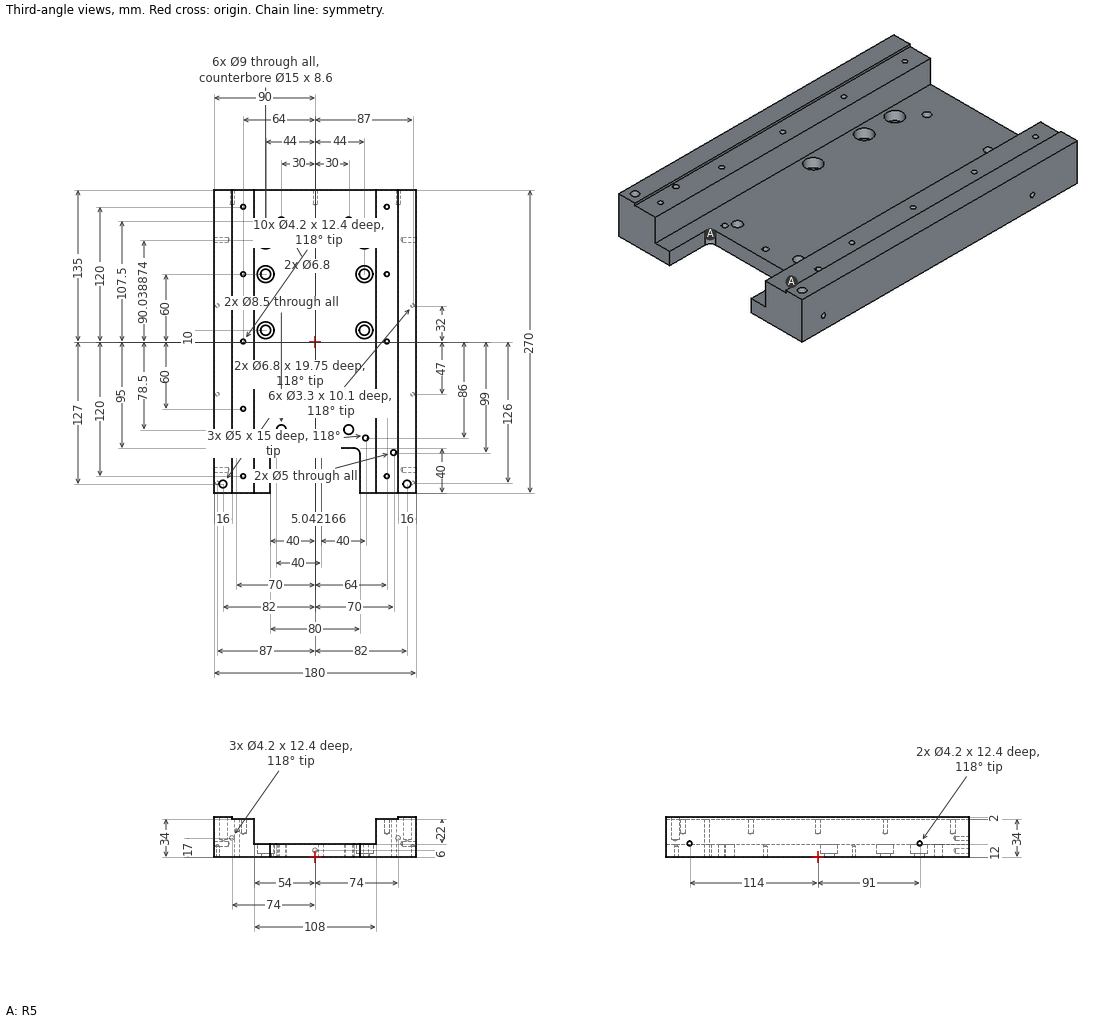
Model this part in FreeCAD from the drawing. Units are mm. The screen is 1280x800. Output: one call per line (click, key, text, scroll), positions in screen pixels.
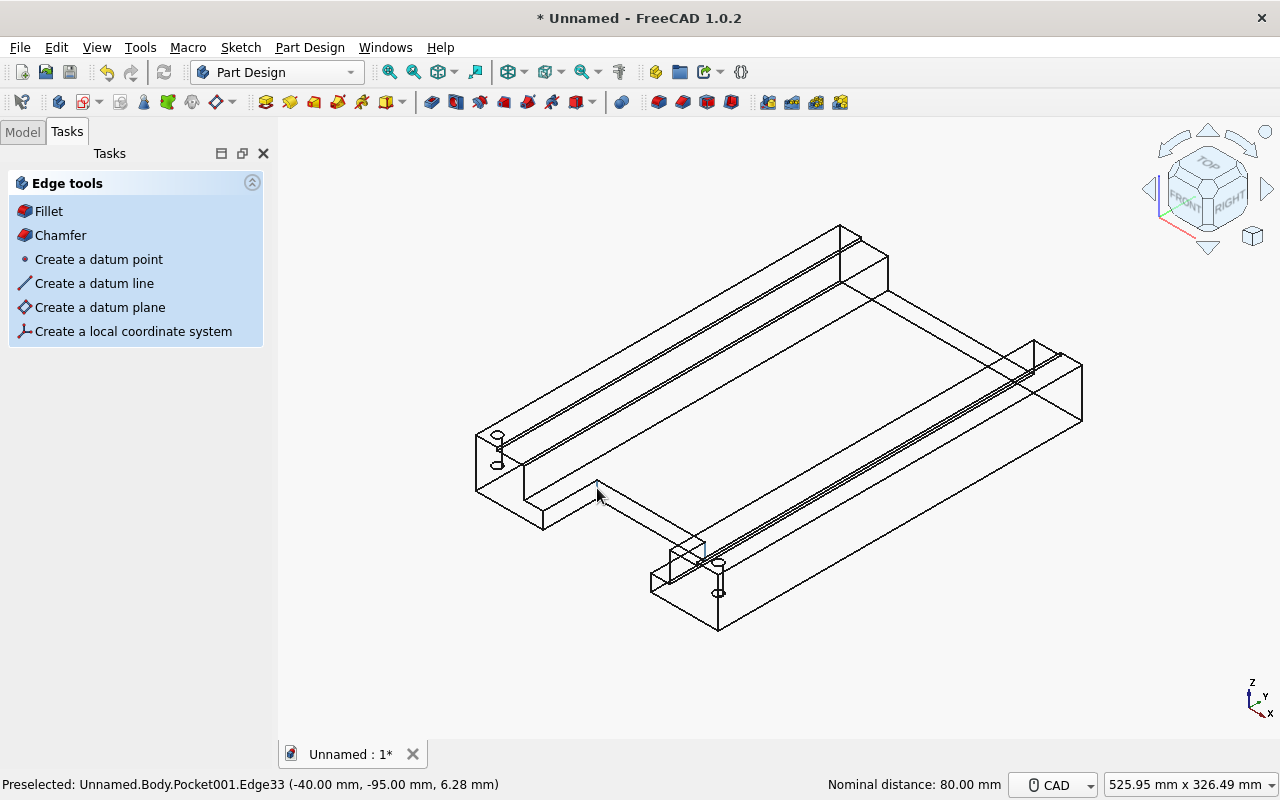
key(v)
key(1)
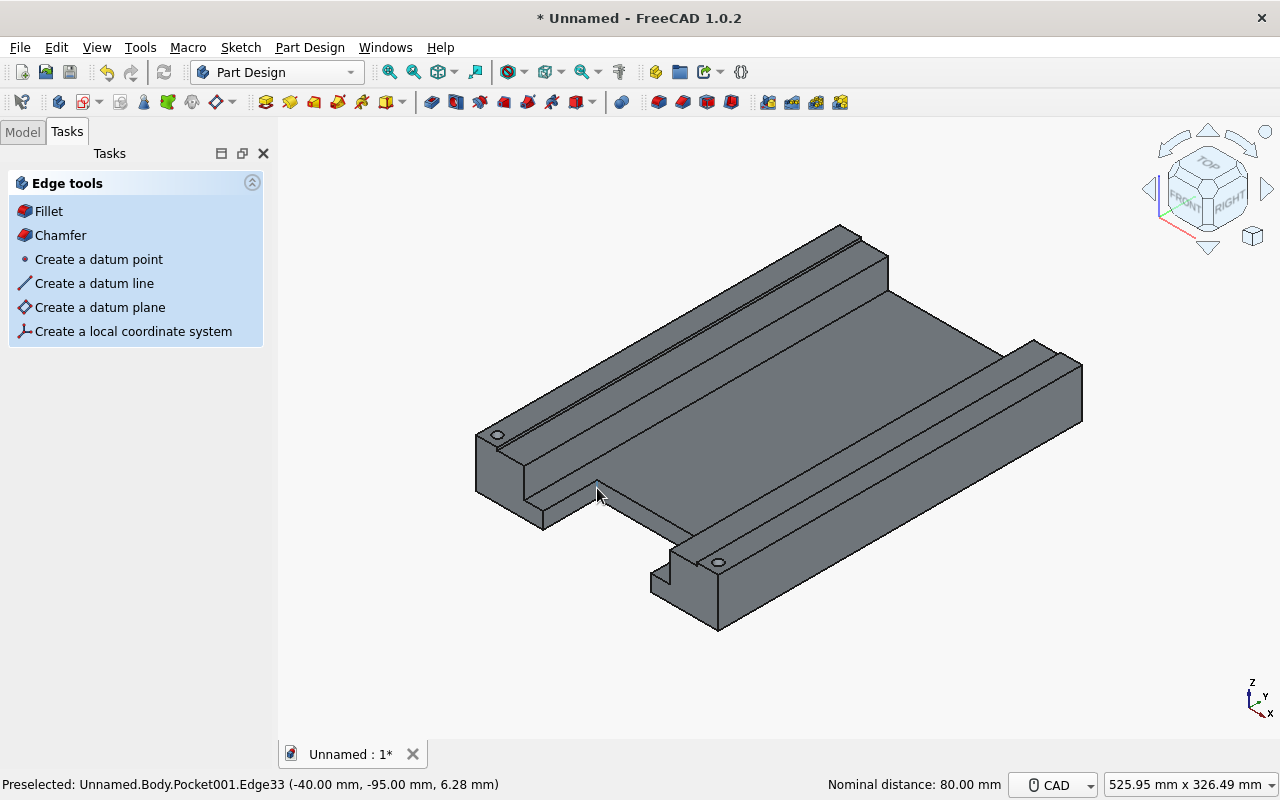
click(660, 102)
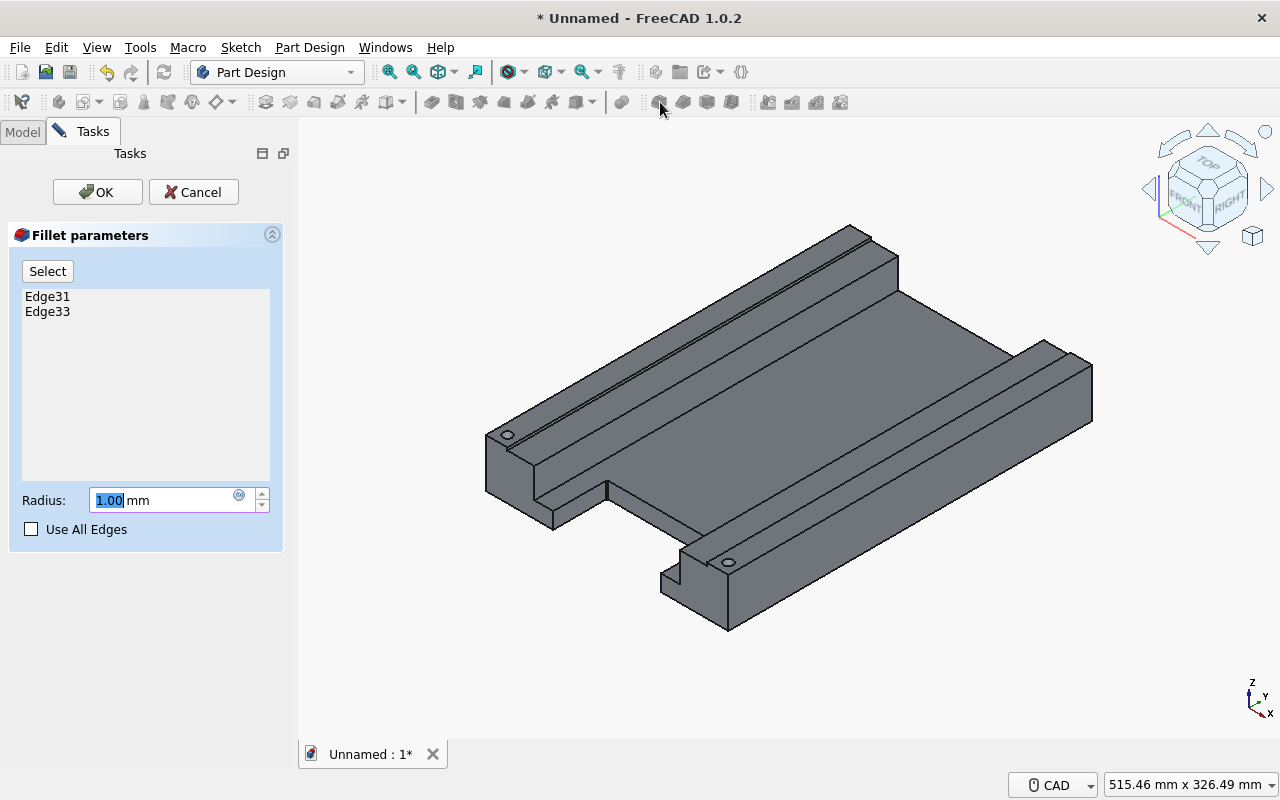
text(5)
key(Tab)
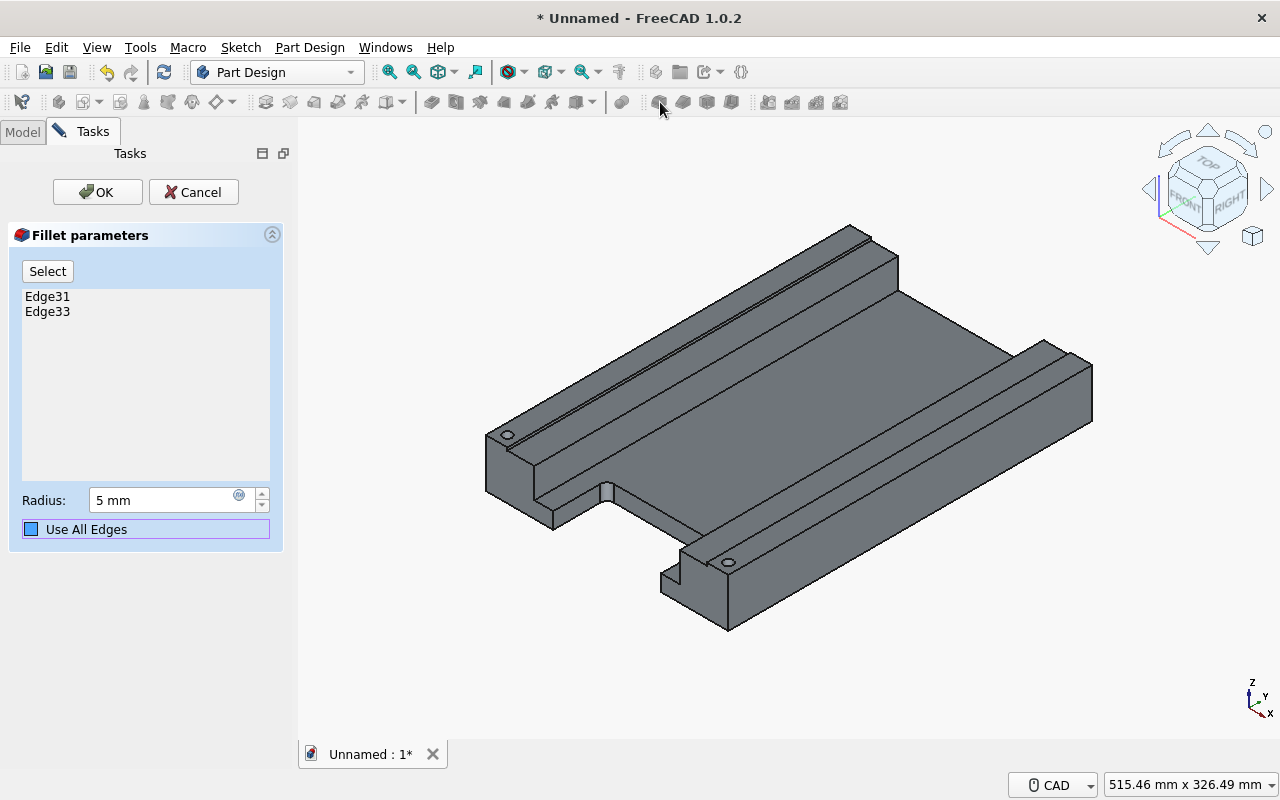
click(98, 192)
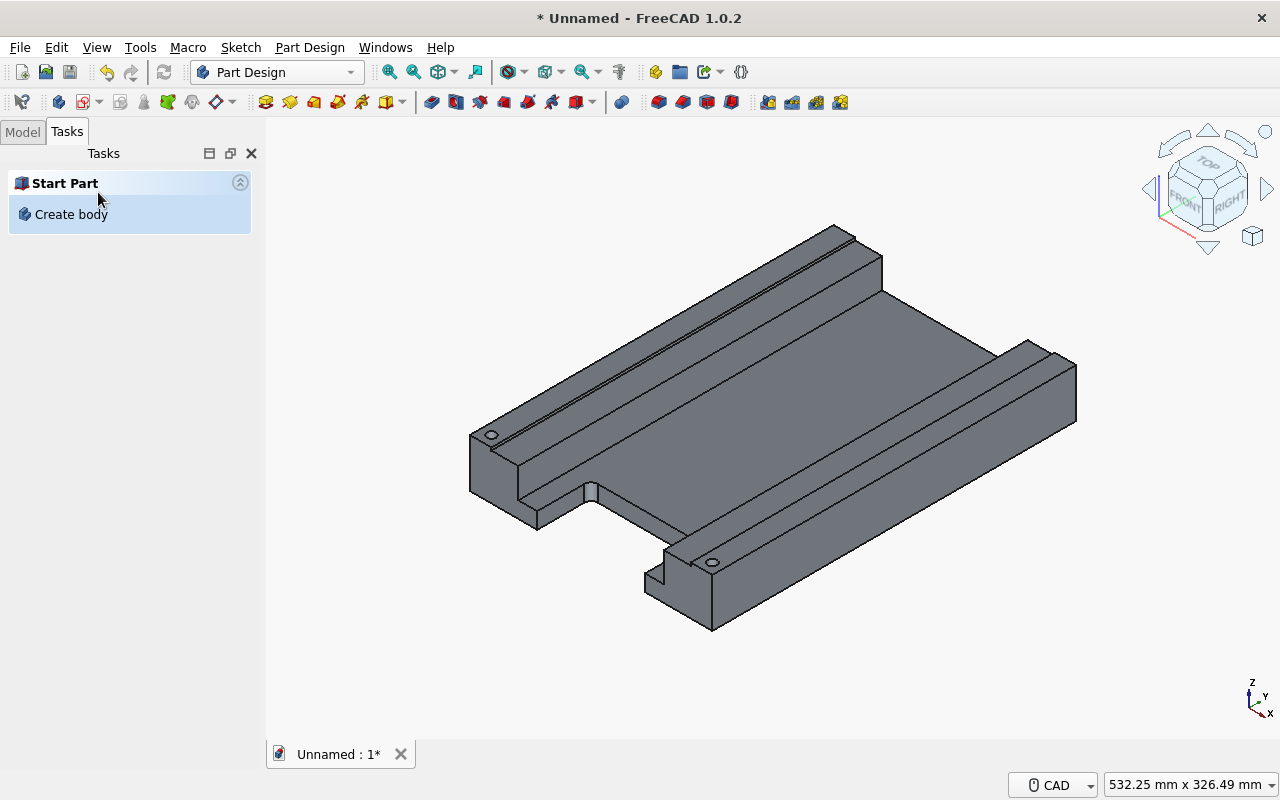
key(4)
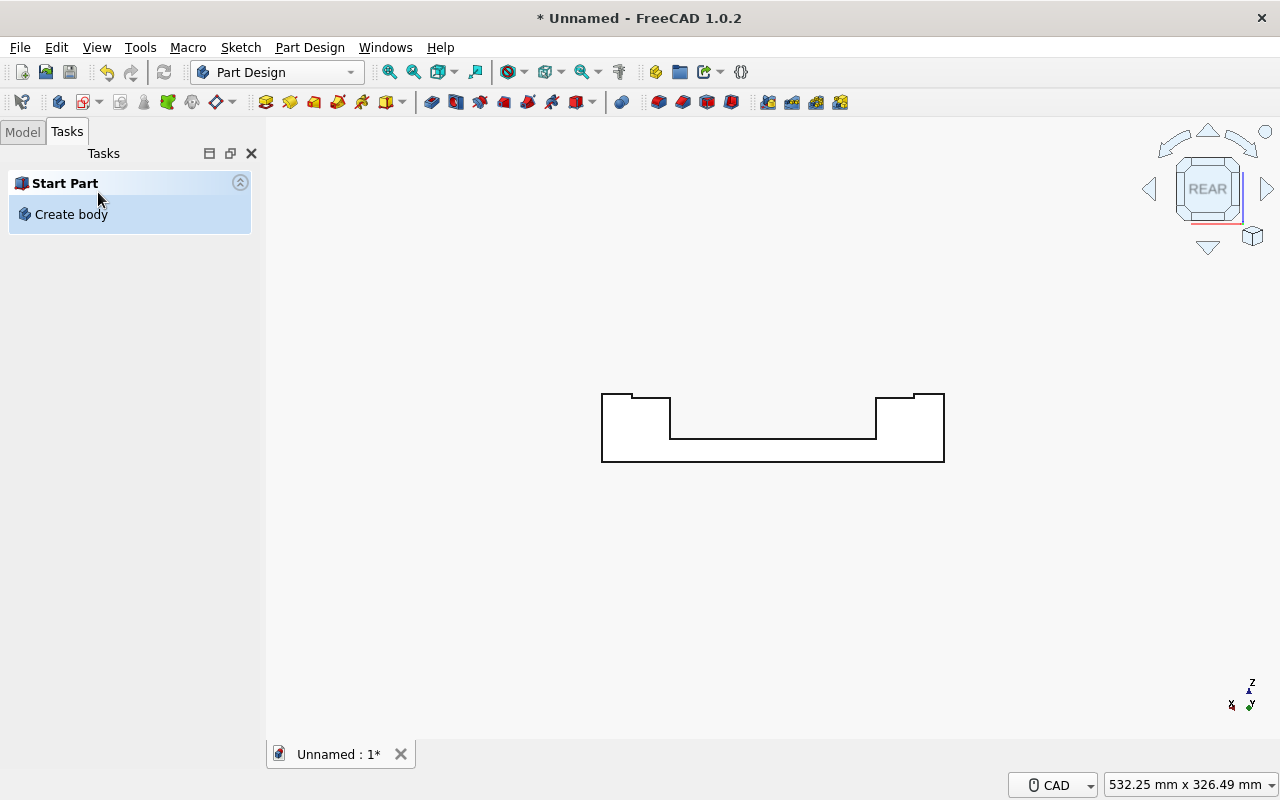
click(390, 72)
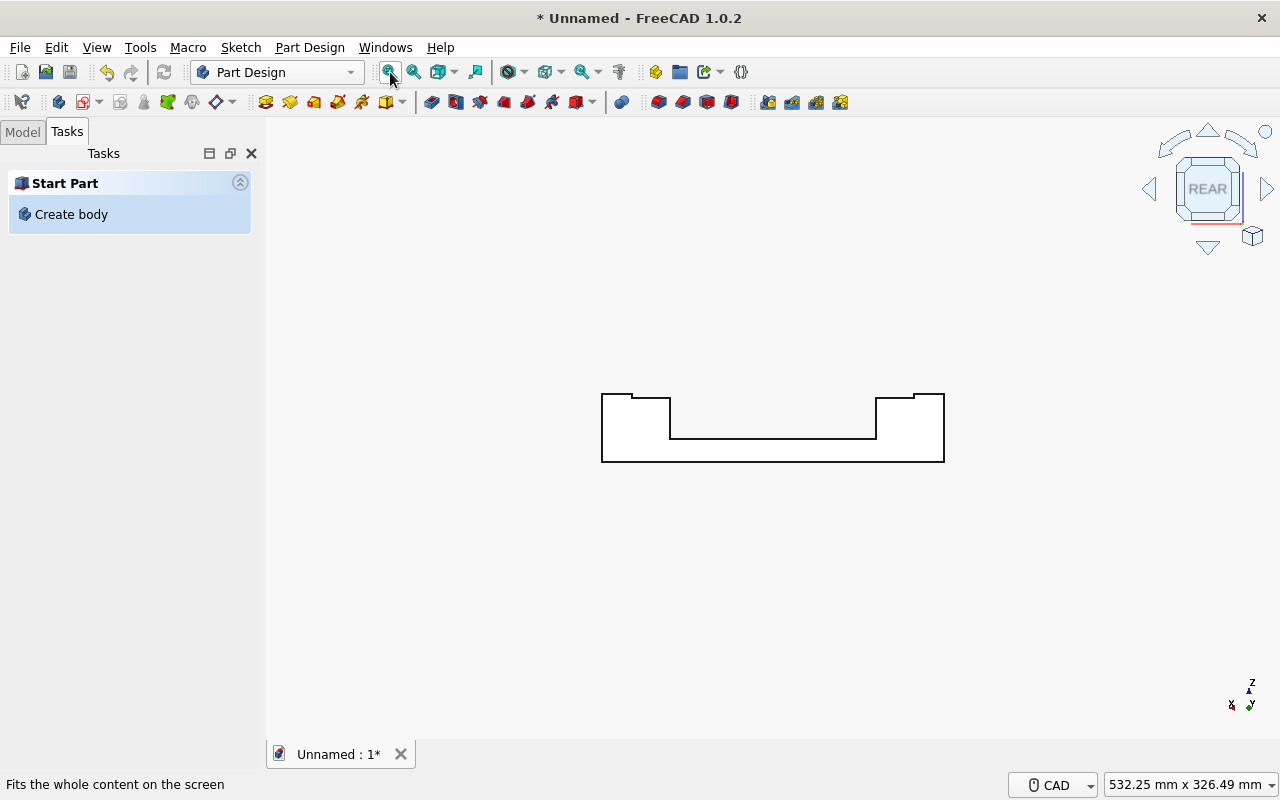
click(626, 427)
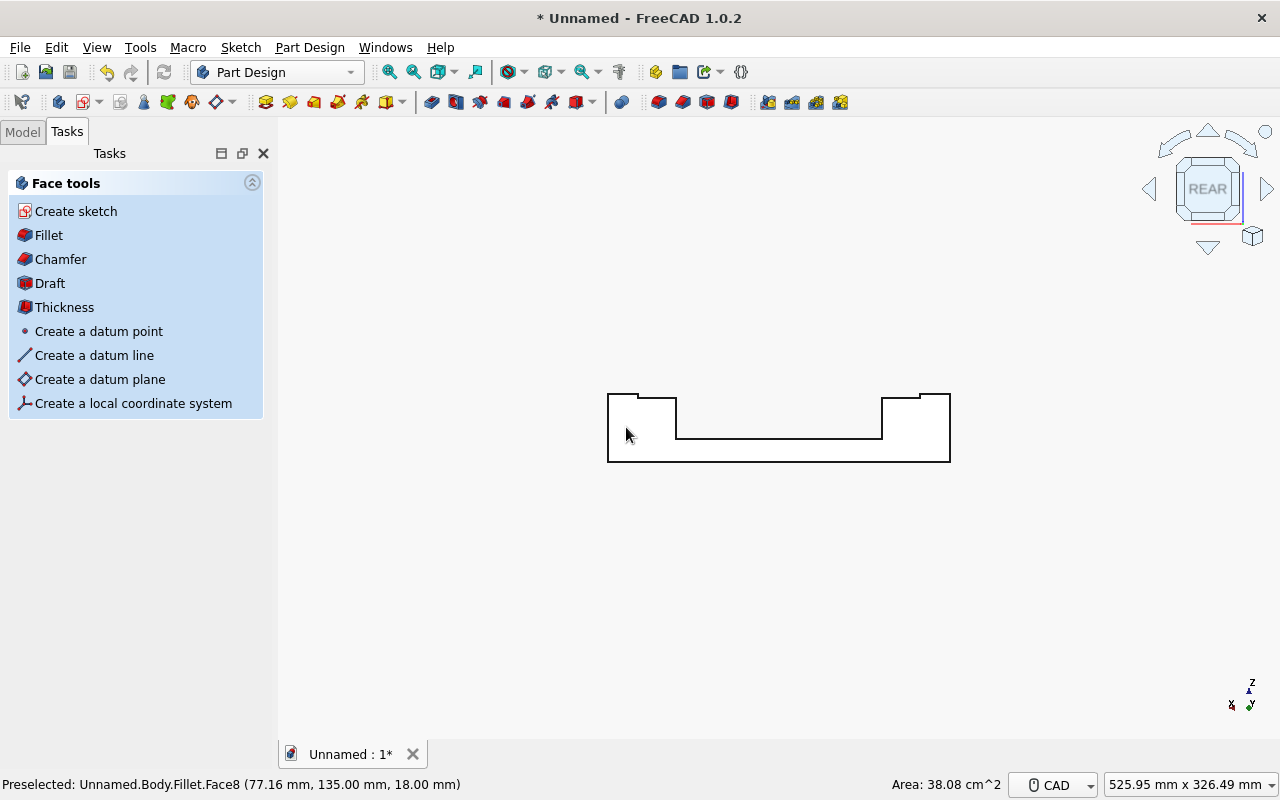
click(84, 102)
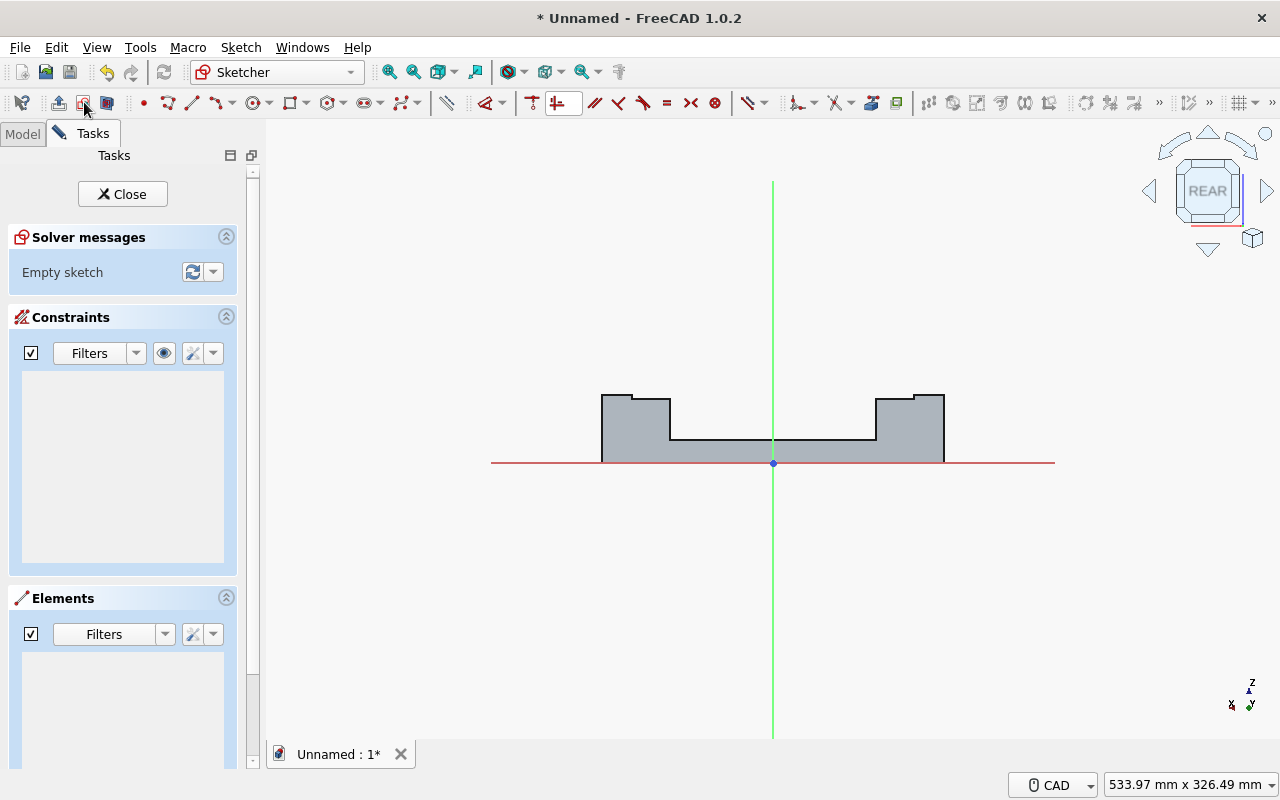
scroll(856, 465, up, 3)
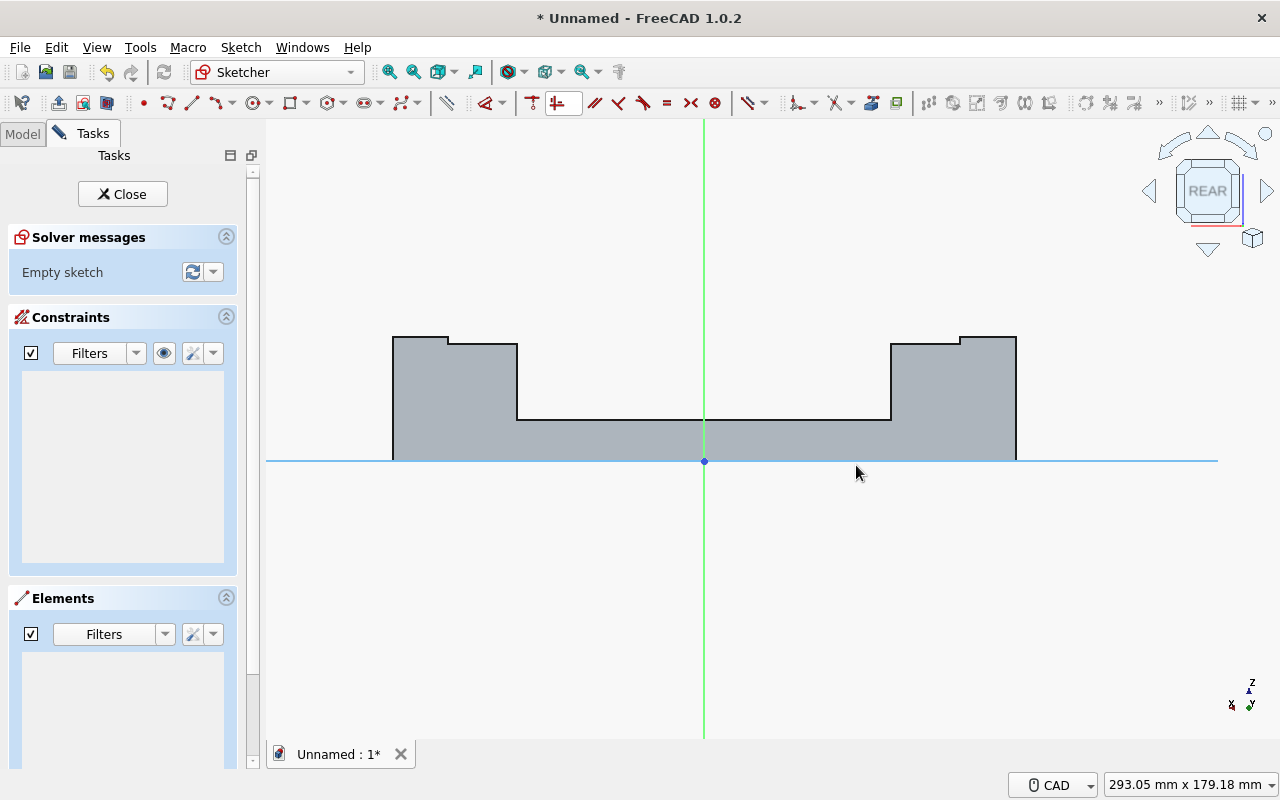
click(254, 104)